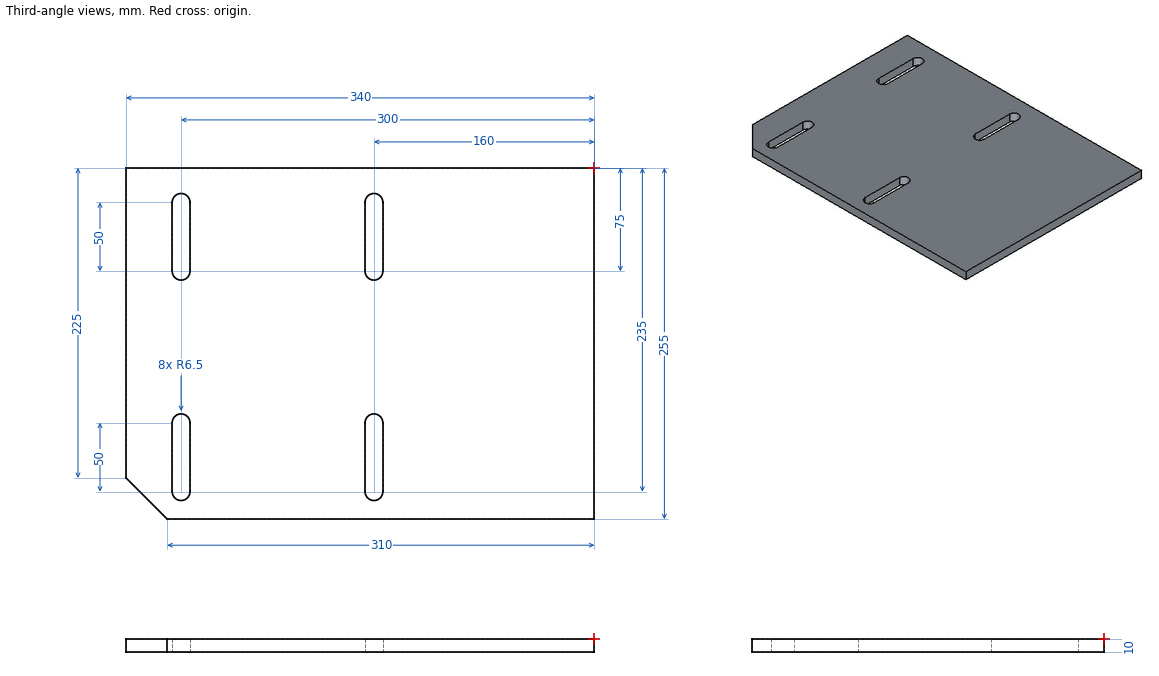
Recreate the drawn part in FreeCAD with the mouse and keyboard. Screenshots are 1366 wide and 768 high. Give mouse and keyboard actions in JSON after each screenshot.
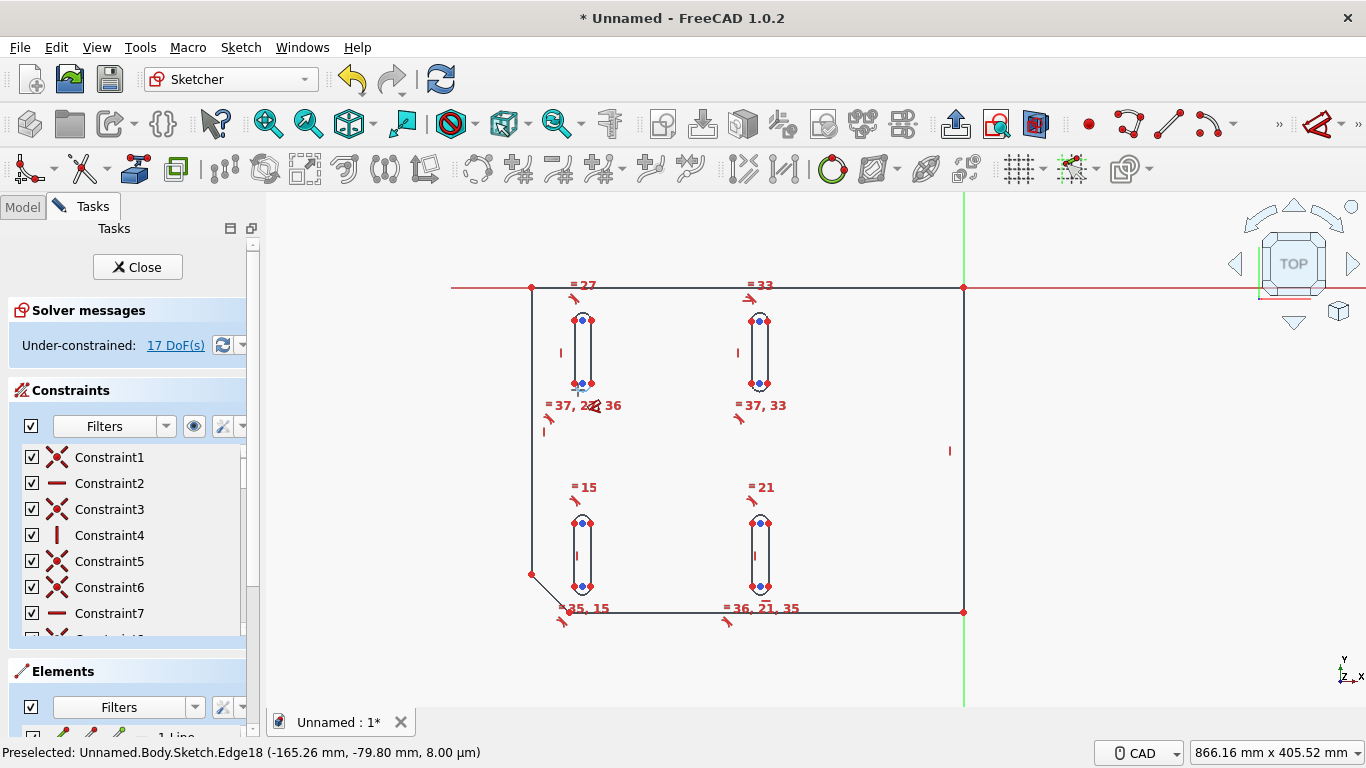
{"action": "scroll", "coordinate": [578, 593], "scroll_direction": "up", "scroll_amount": 8}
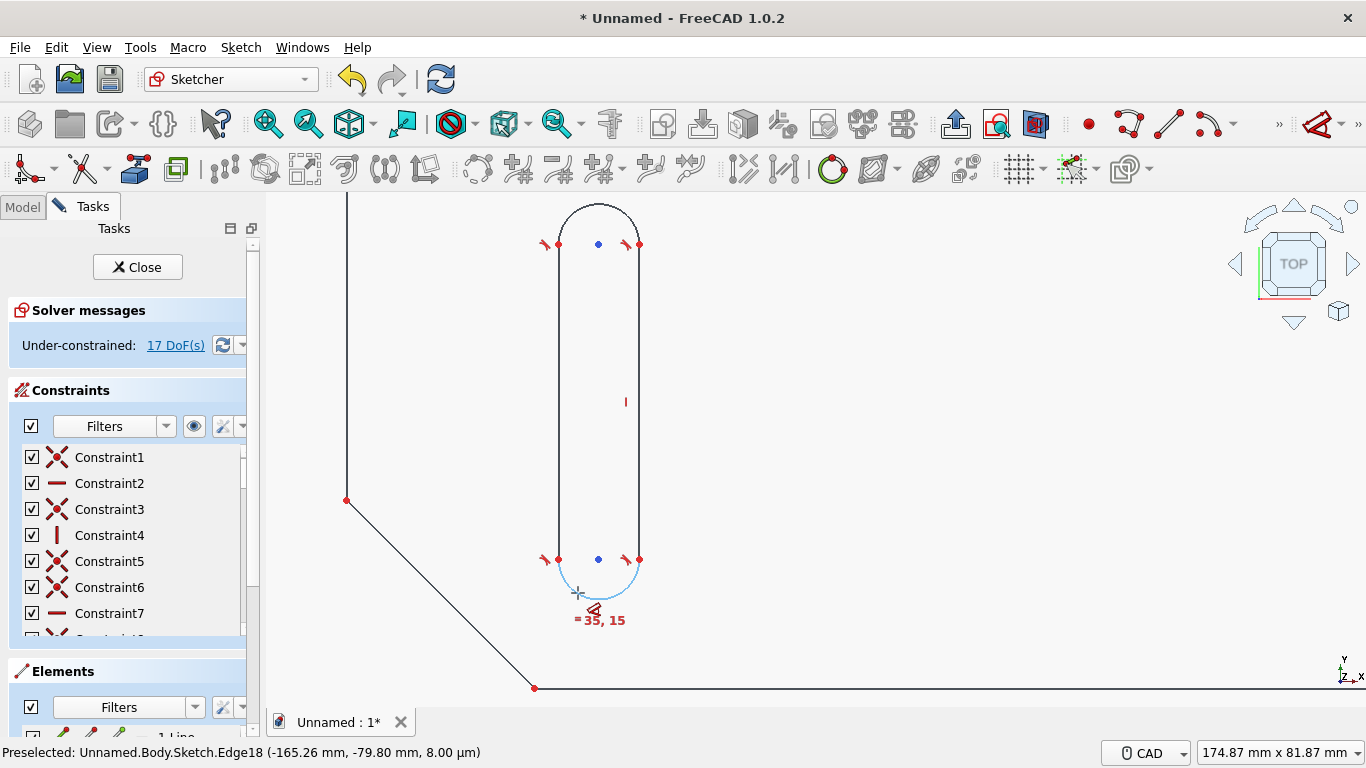
{"action": "left_click", "coordinate": [575, 592]}
{"action": "left_click", "coordinate": [556, 618]}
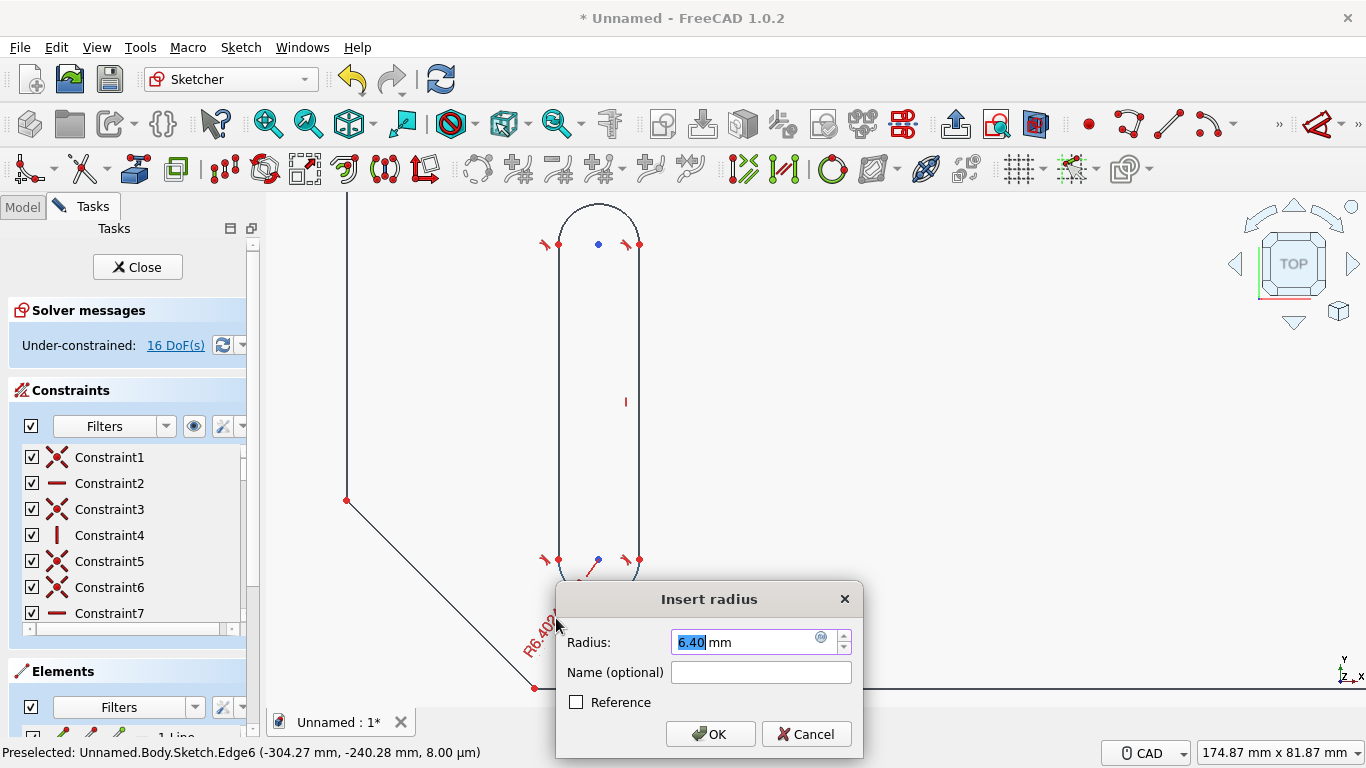
{"action": "type", "text": "6.5"}
{"action": "key", "text": "Return"}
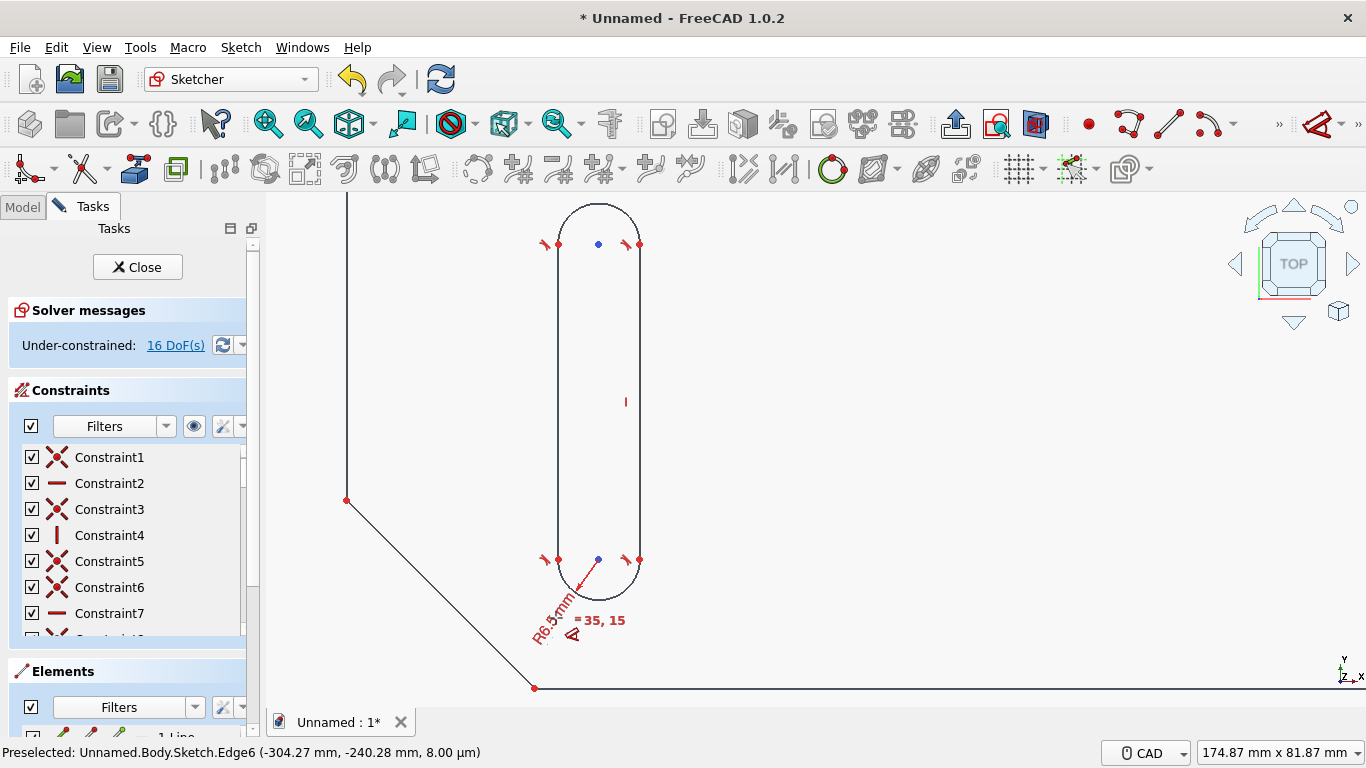
{"action": "scroll", "coordinate": [578, 593], "scroll_direction": "down", "scroll_amount": 8}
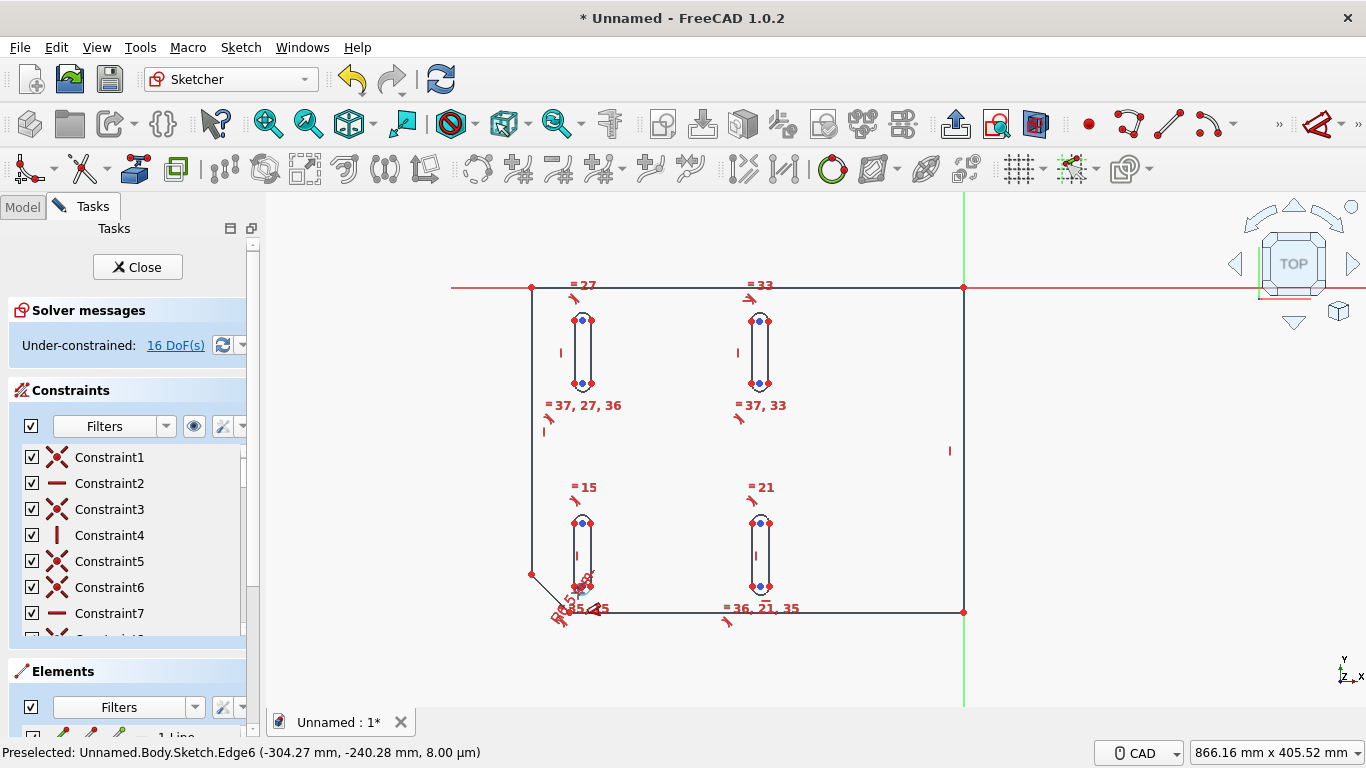
{"action": "left_click", "coordinate": [574, 568]}
{"action": "left_click", "coordinate": [608, 555]}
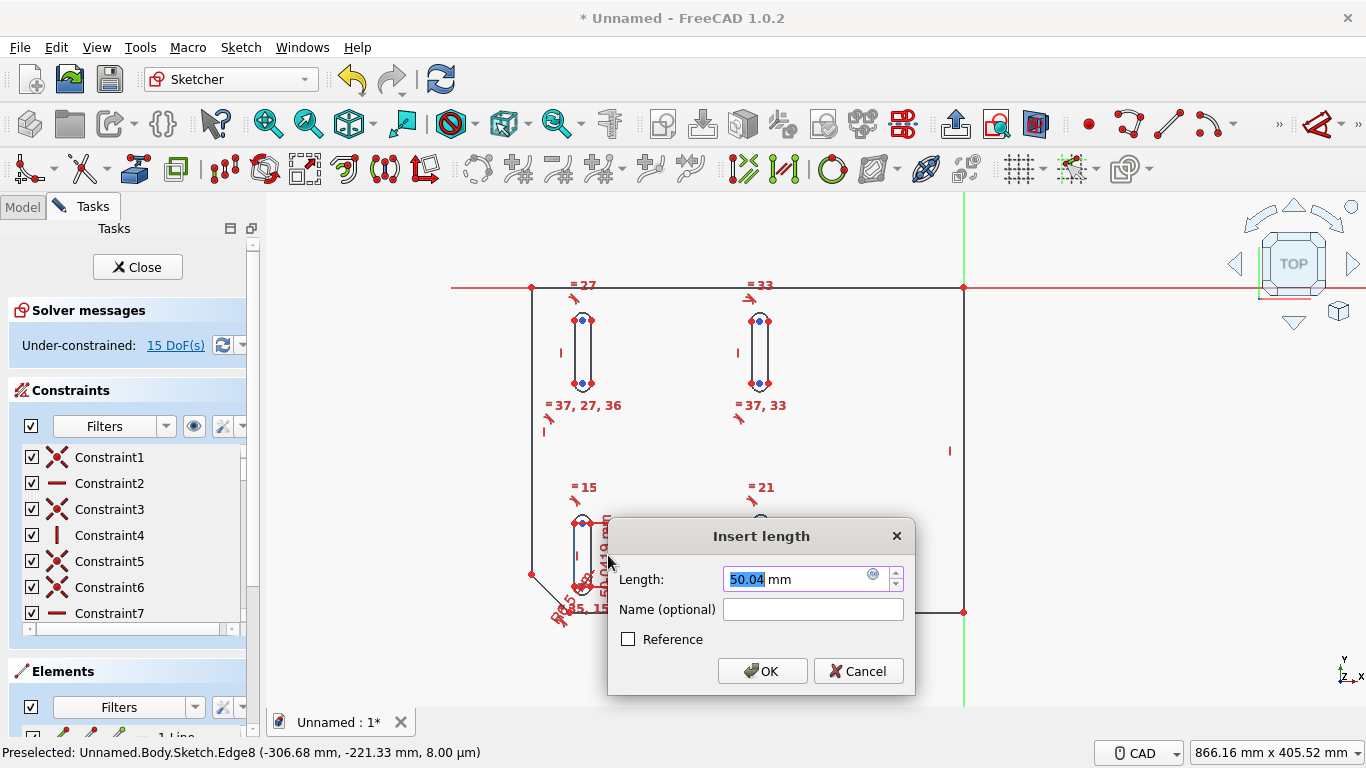
{"action": "type", "text": "50"}
{"action": "key", "text": "Return"}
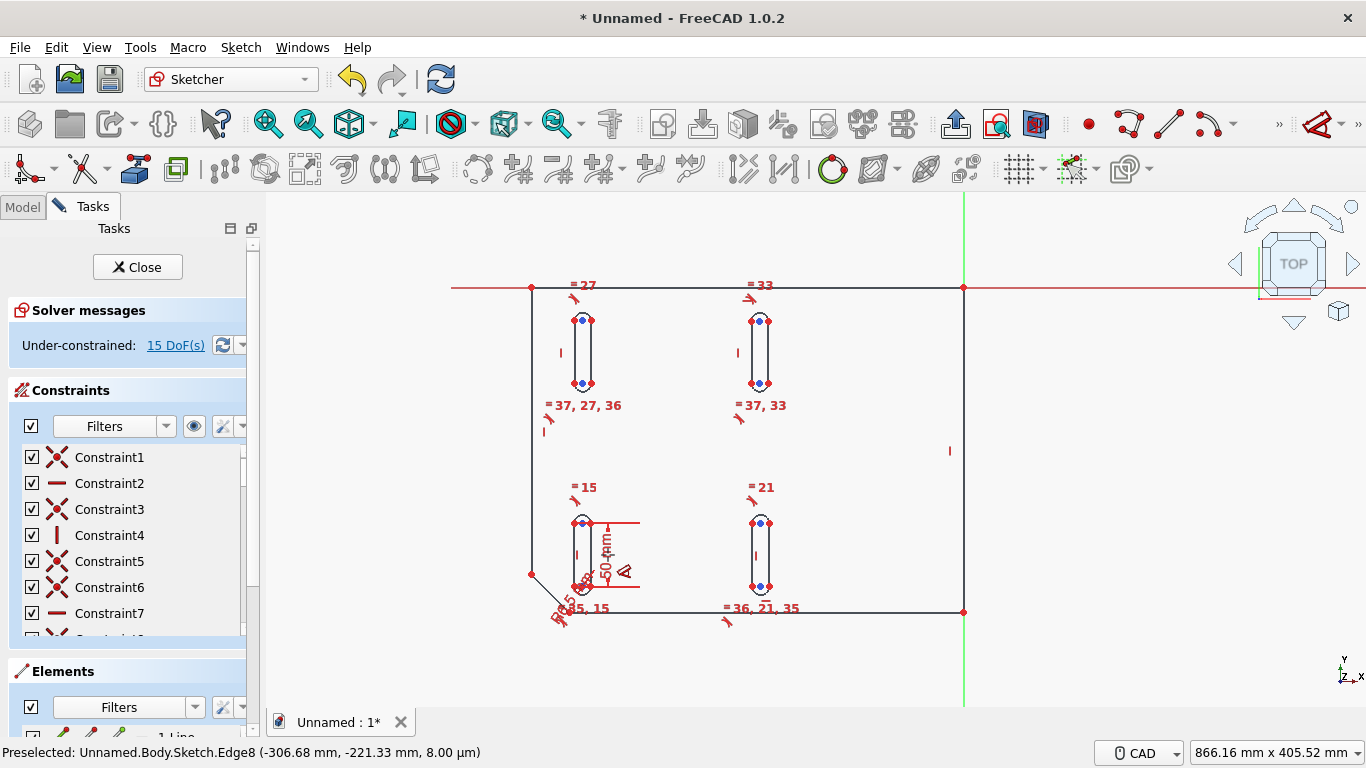
{"action": "left_click", "coordinate": [753, 568]}
{"action": "left_click", "coordinate": [787, 555]}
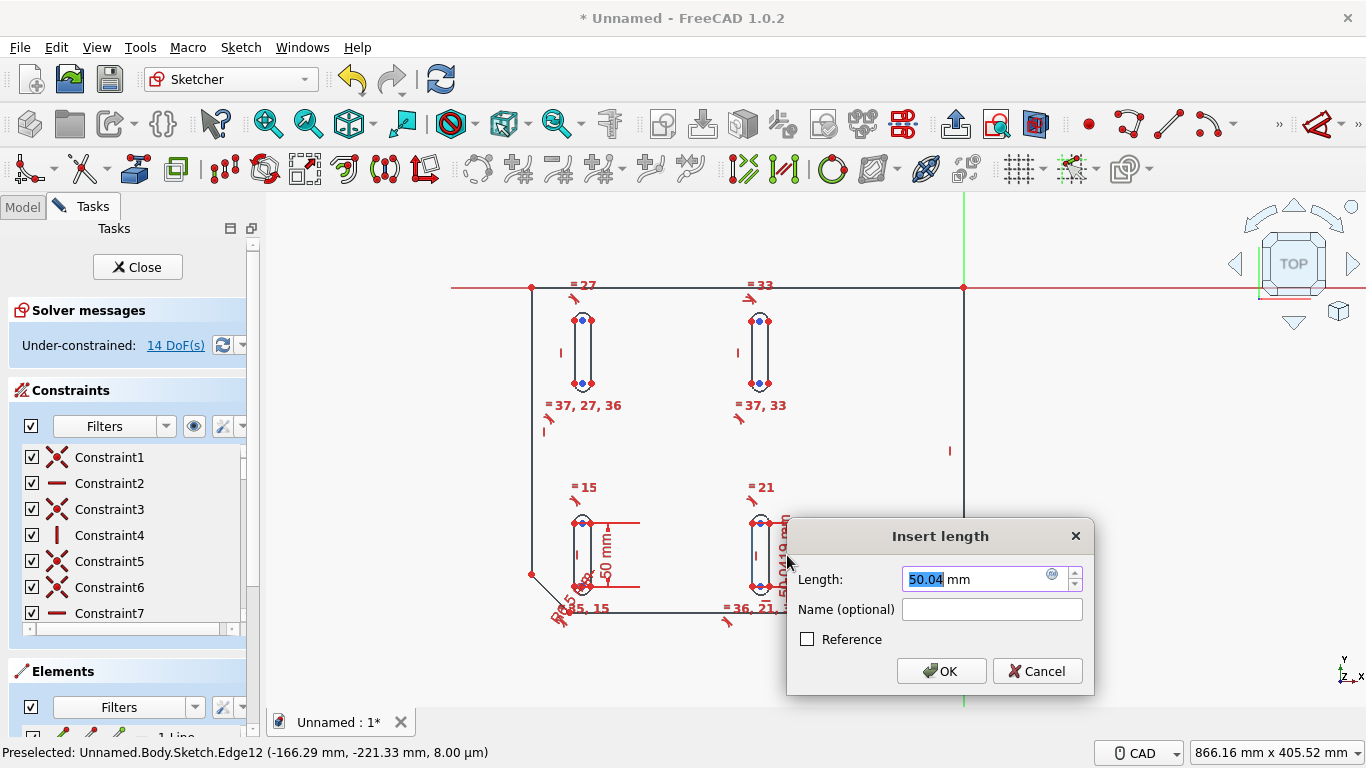
{"action": "type", "text": "50"}
{"action": "key", "text": "Return"}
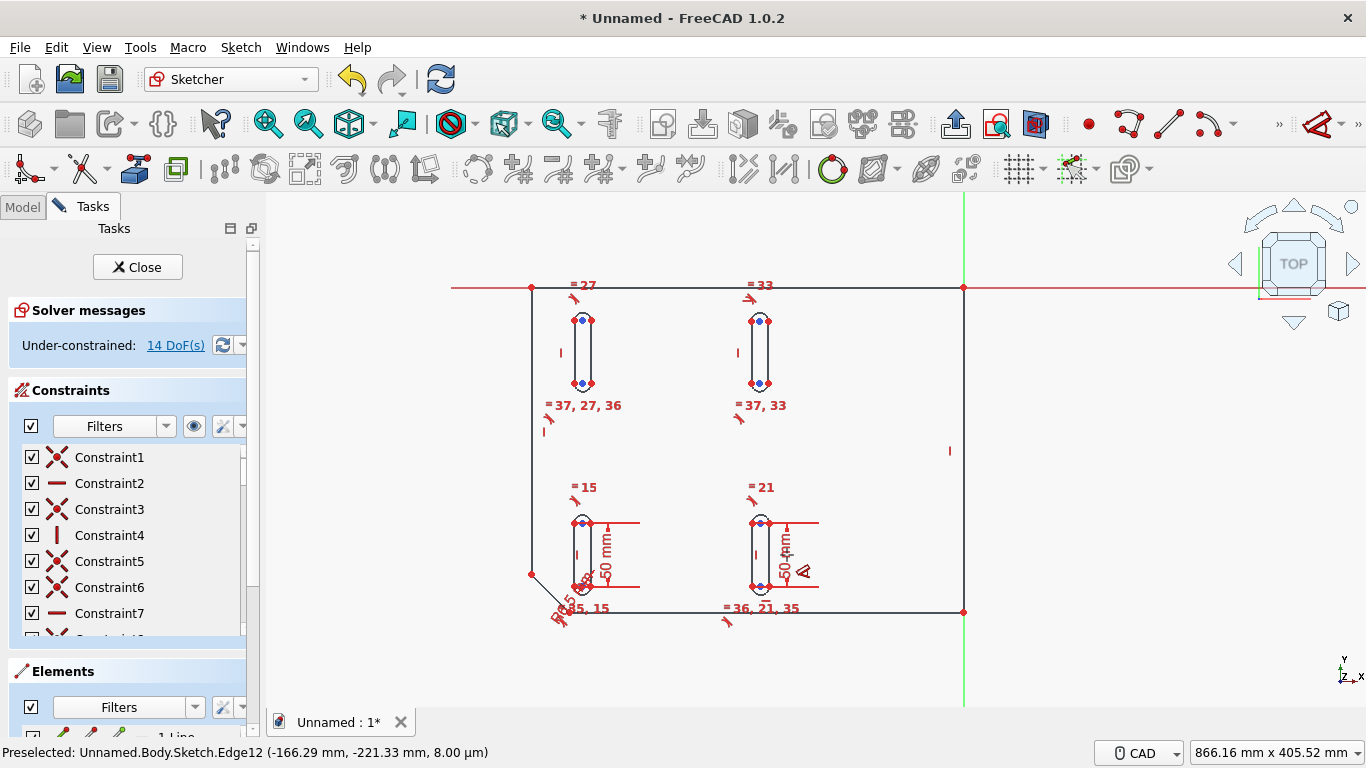
{"action": "left_click", "coordinate": [575, 365]}
{"action": "left_click", "coordinate": [609, 352]}